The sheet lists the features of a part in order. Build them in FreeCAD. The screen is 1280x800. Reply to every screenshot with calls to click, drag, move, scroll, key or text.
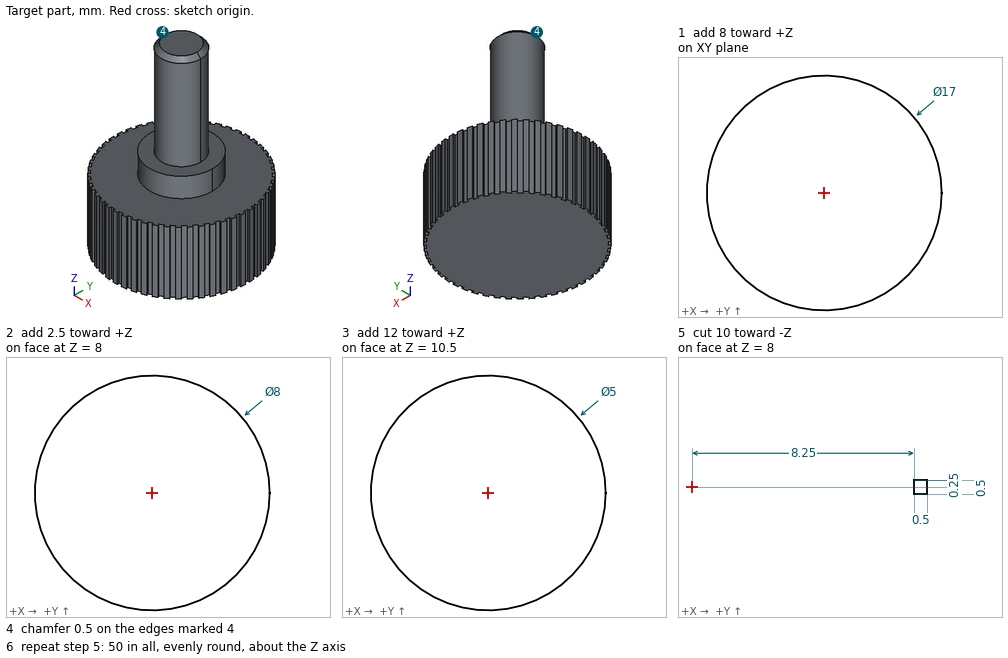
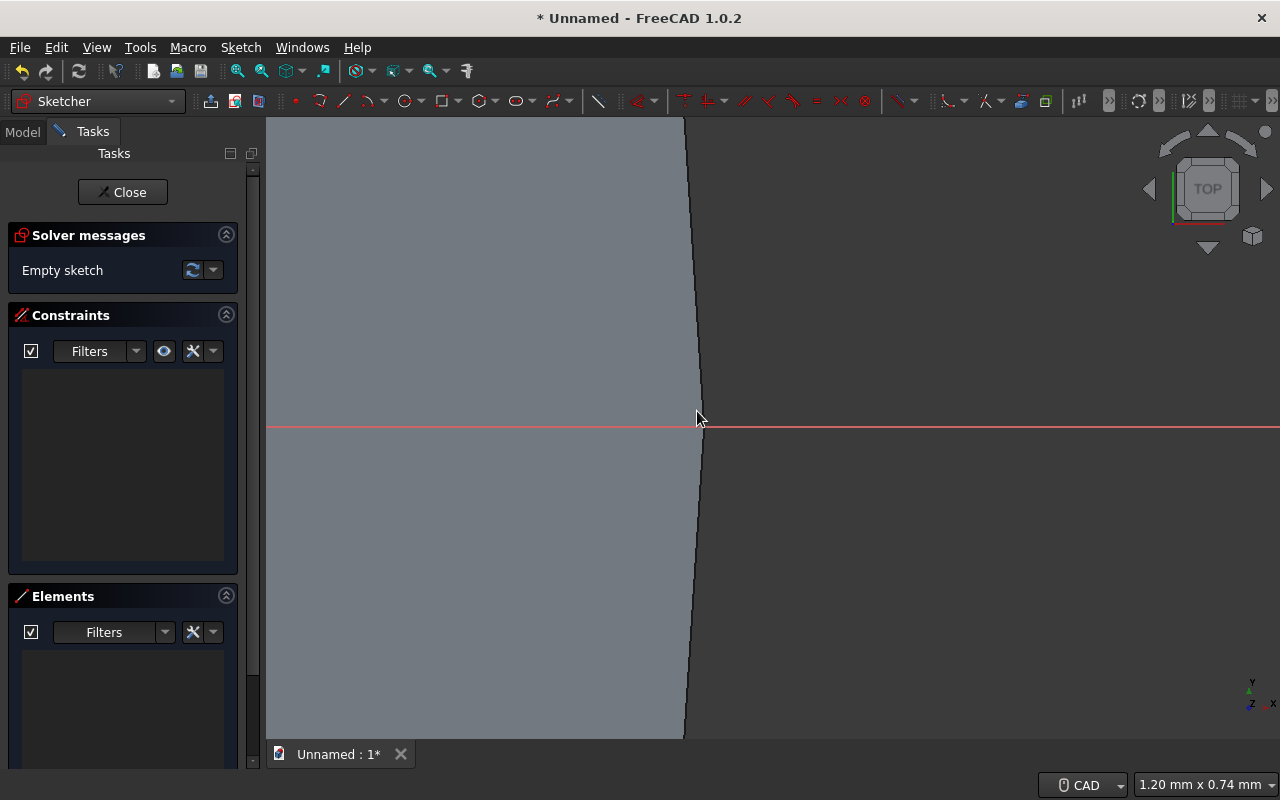
key(g)
key(r)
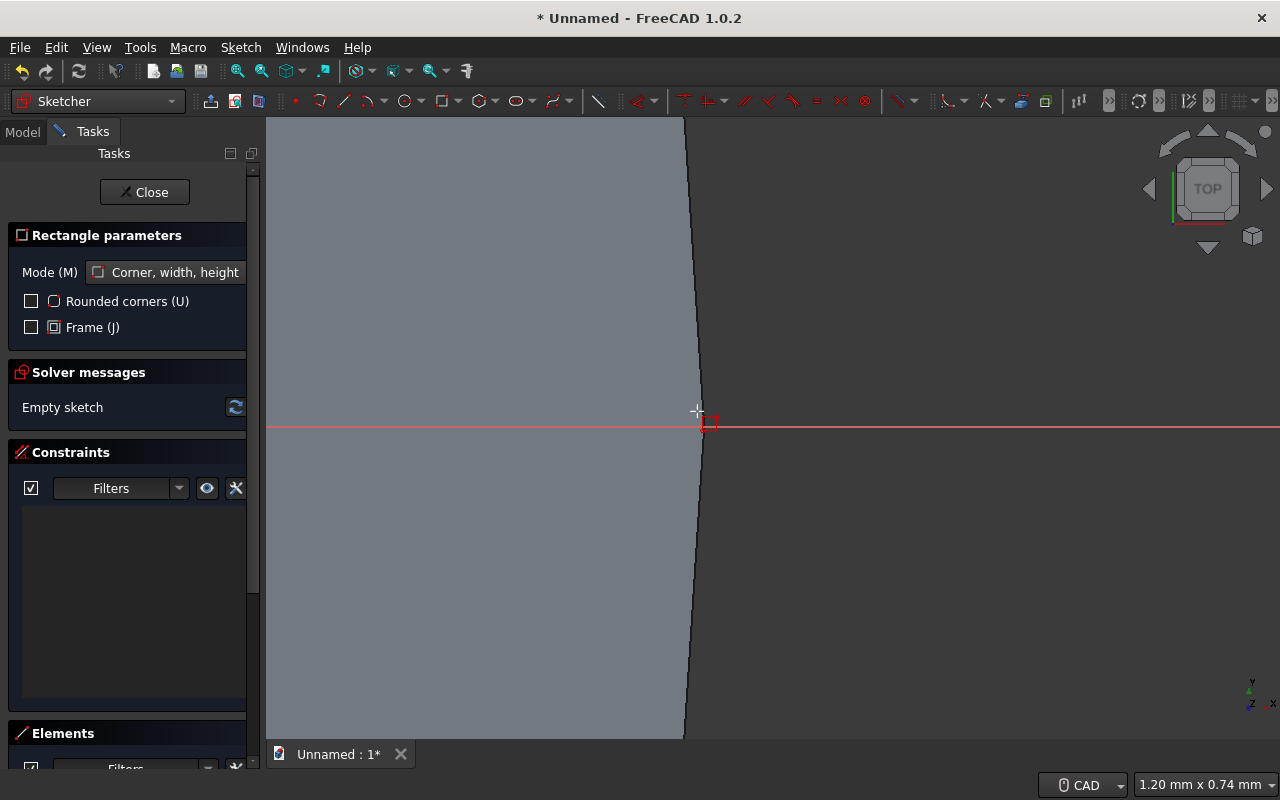
click(493, 216)
click(915, 638)
key(Escape)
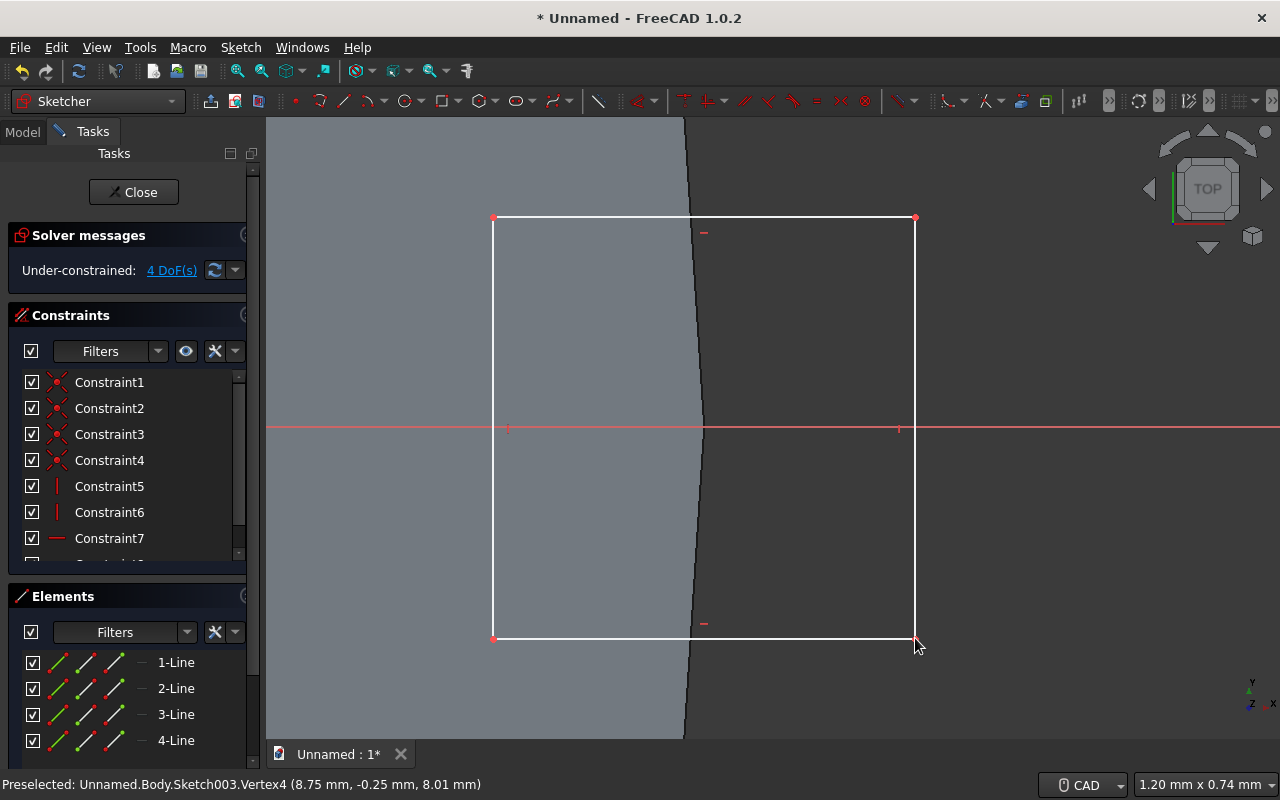
key(d)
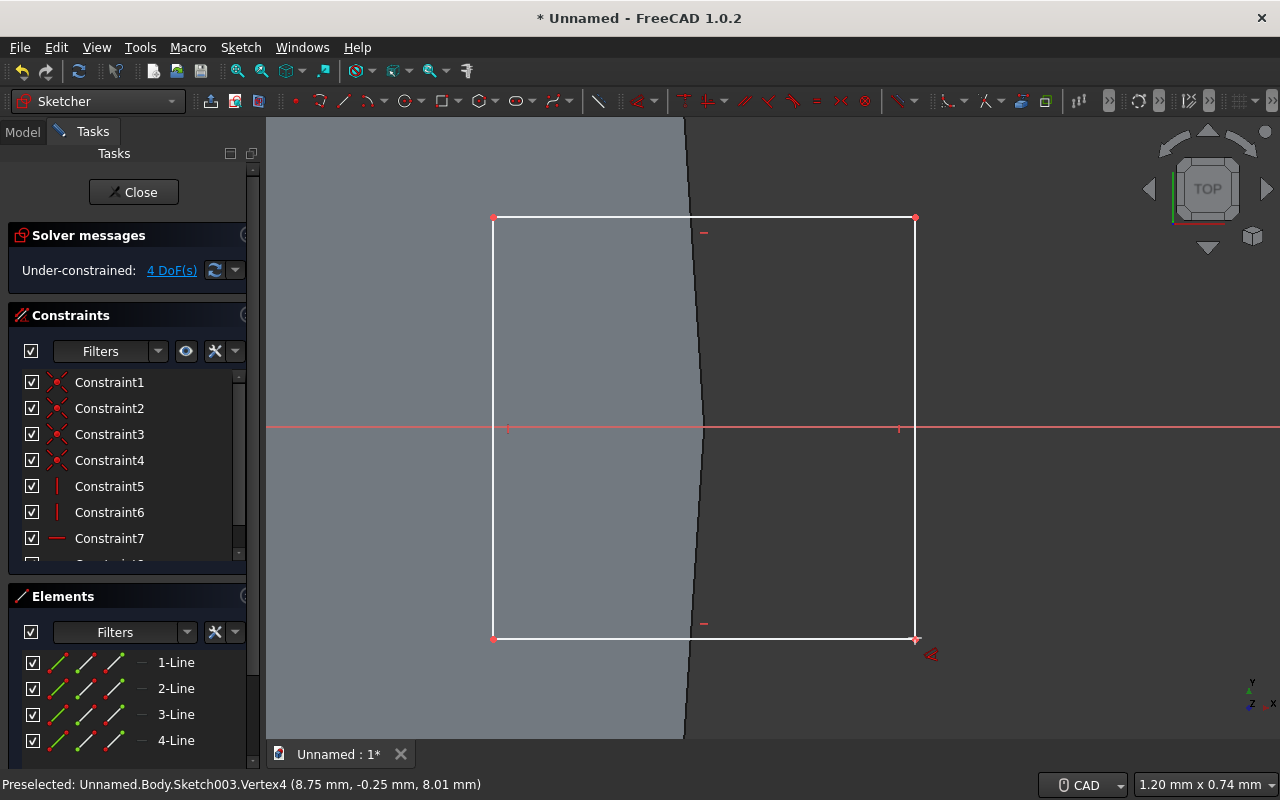
click(493, 344)
click(459, 331)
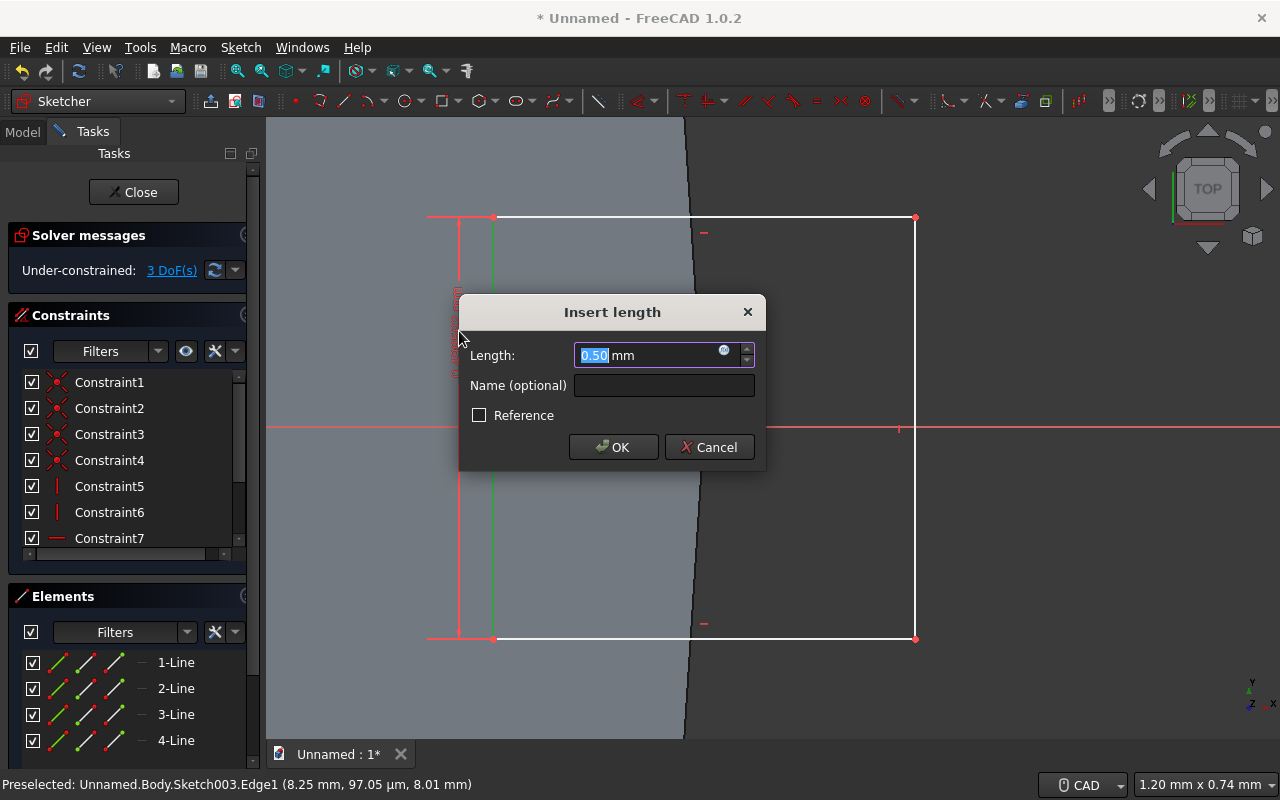
text(0.5)
key(Return)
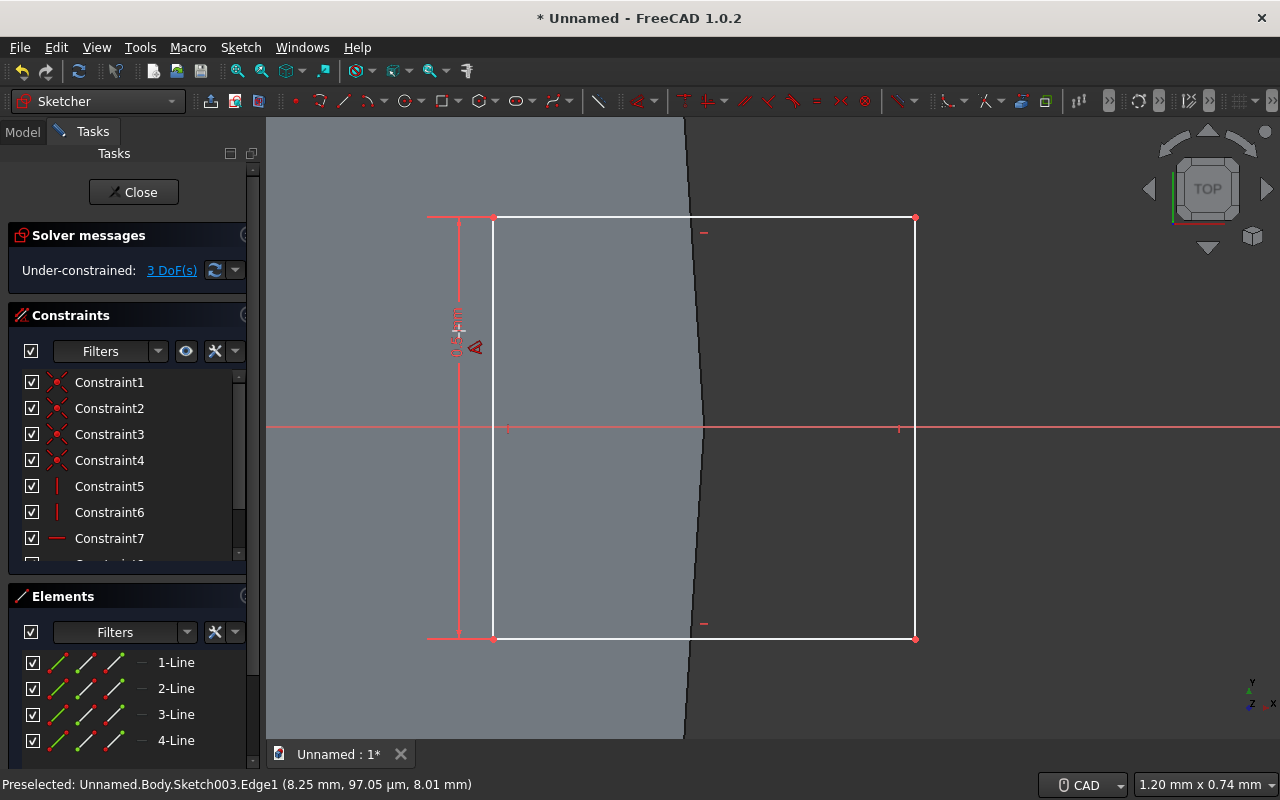
click(620, 639)
click(704, 673)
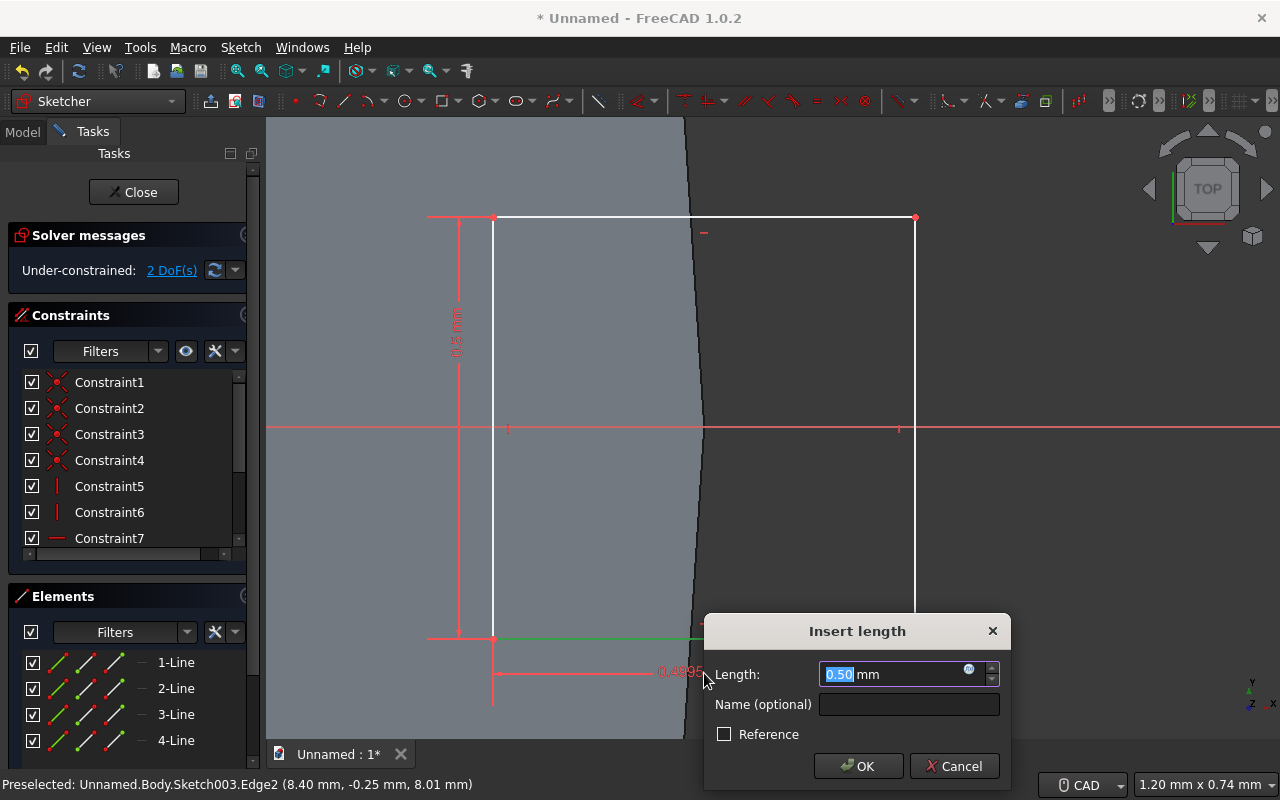
text(0.5)
key(Return)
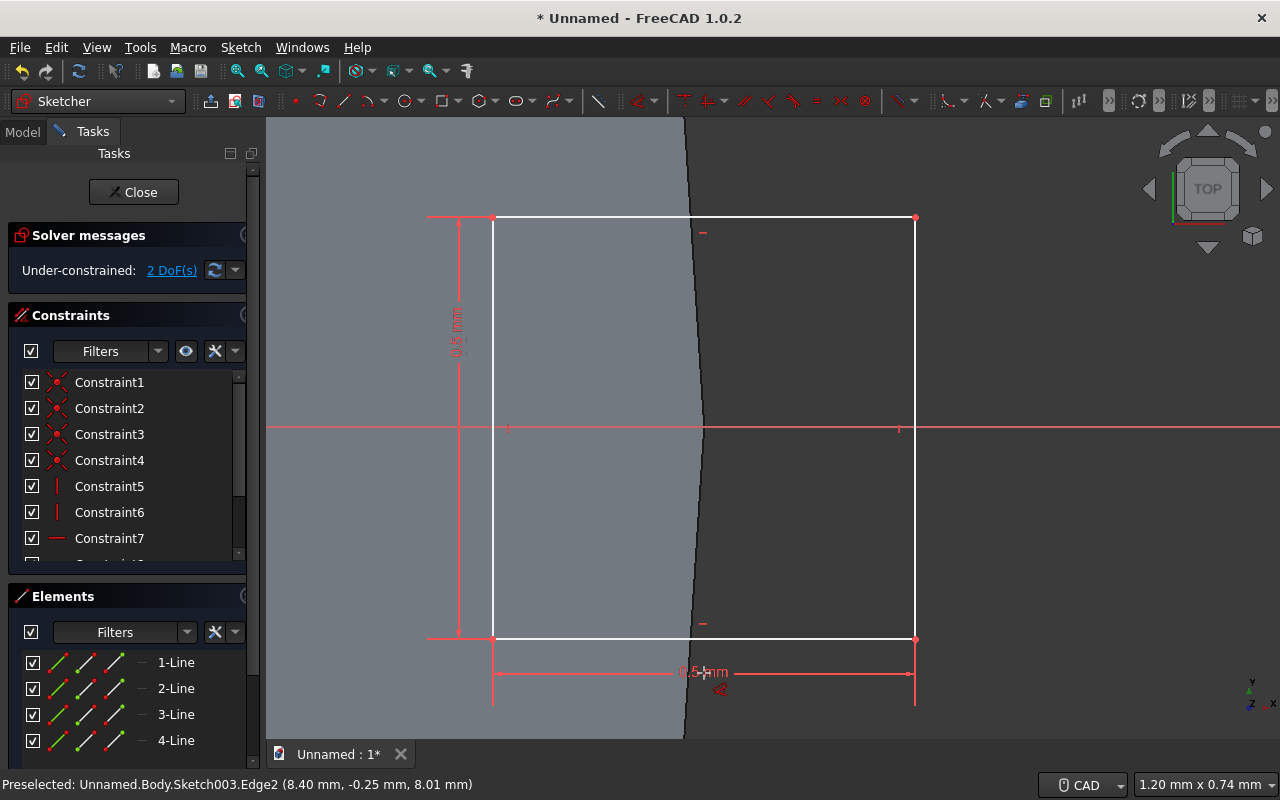
click(493, 217)
click(393, 183)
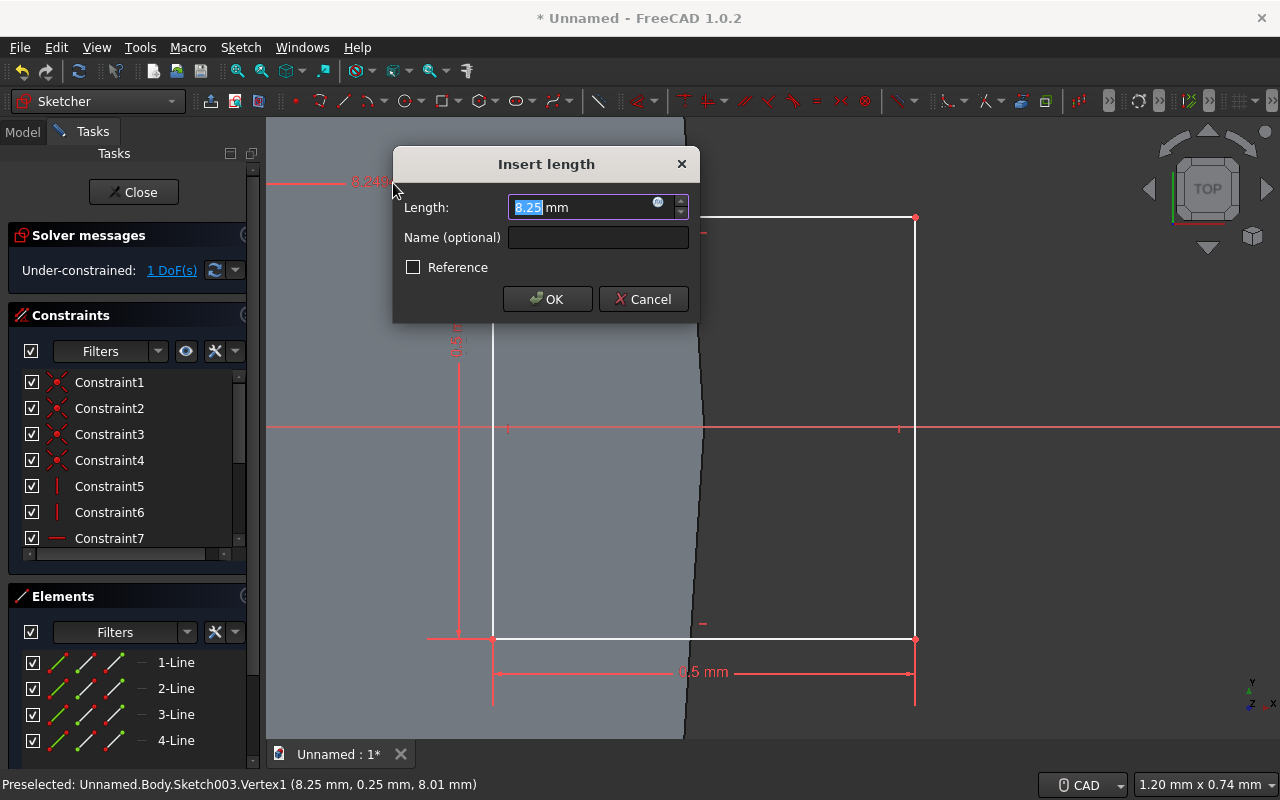
text(8.25)
key(Return)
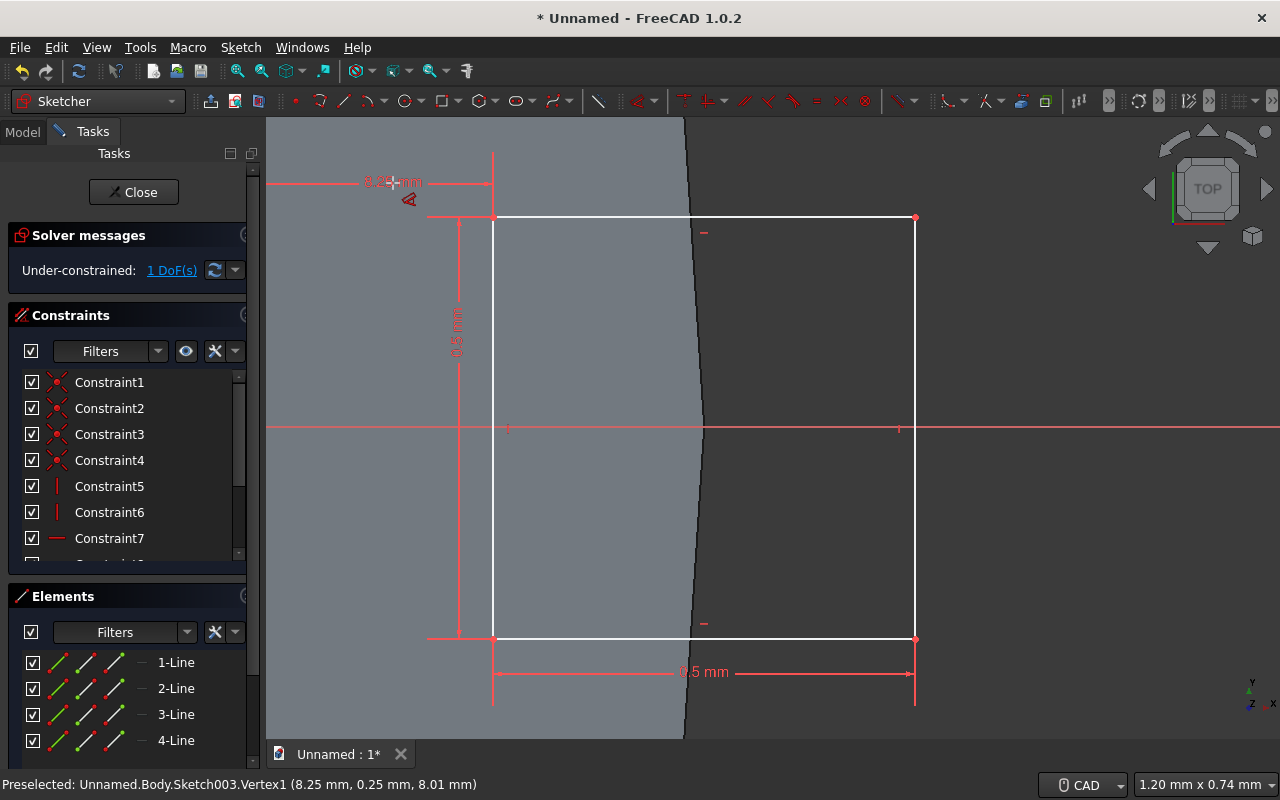
click(493, 217)
click(527, 274)